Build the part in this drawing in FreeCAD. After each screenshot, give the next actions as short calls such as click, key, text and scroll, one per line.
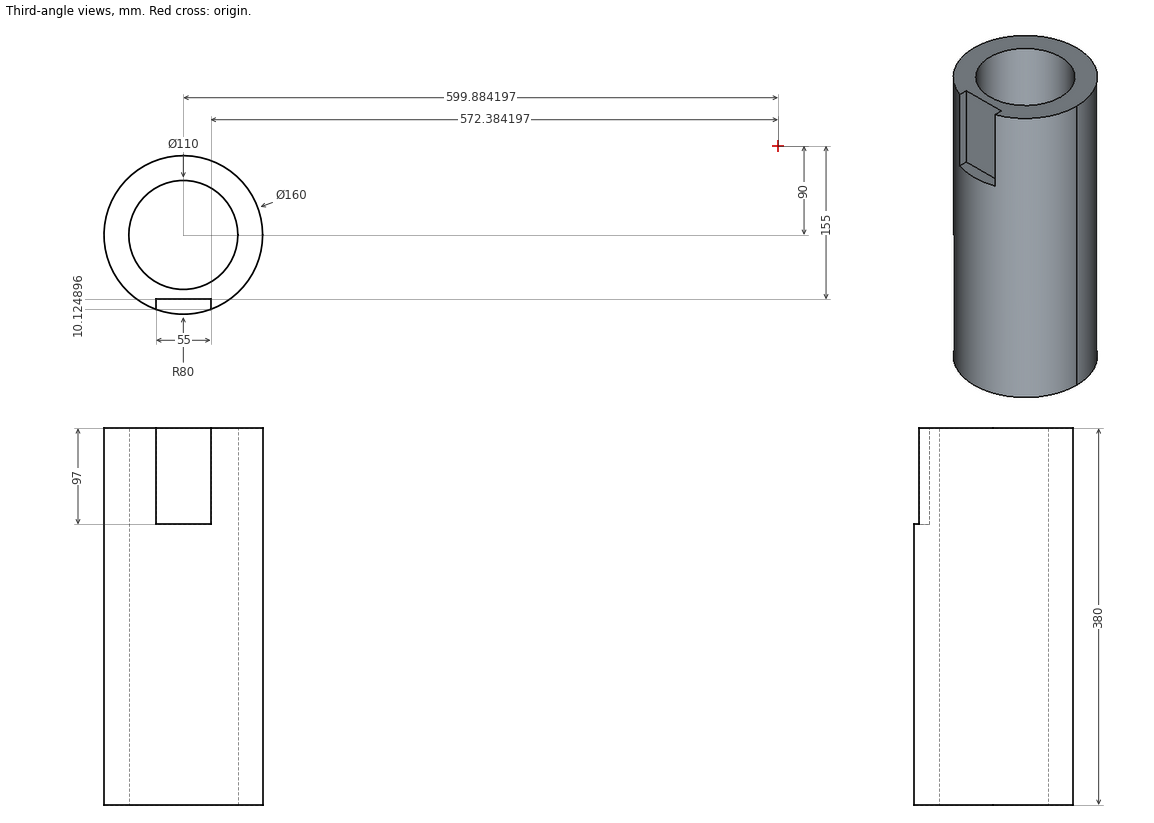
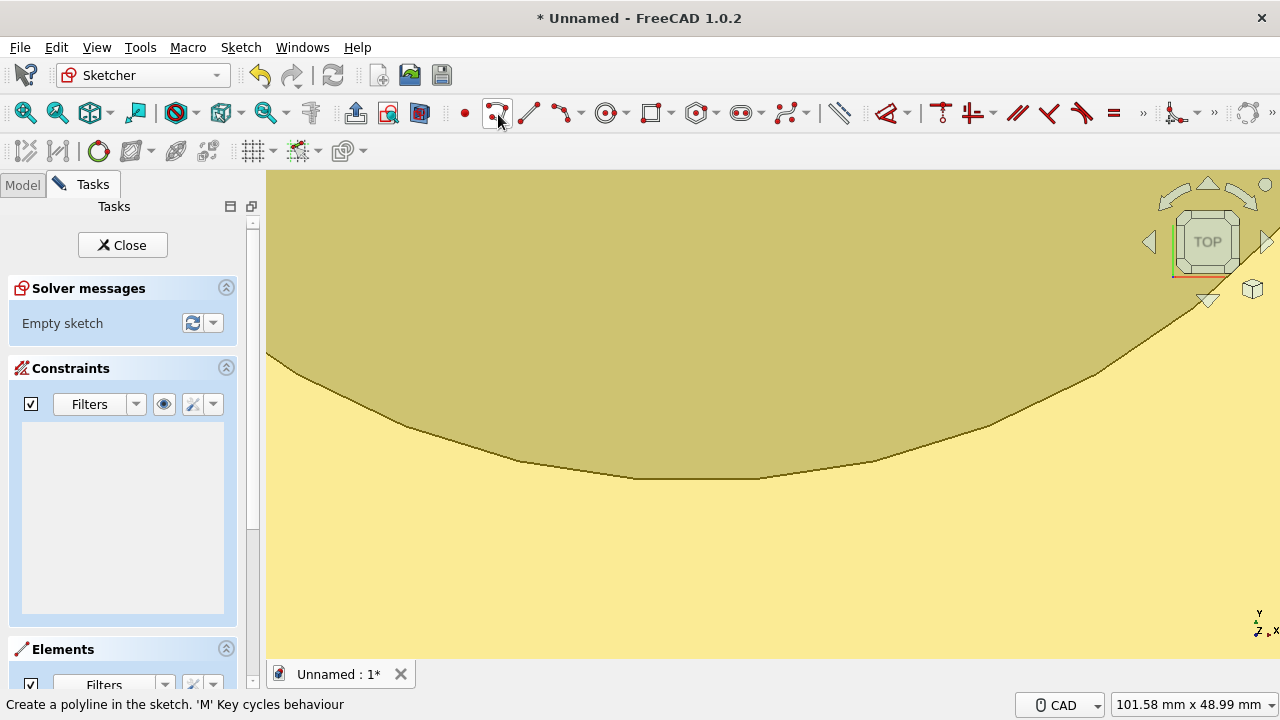
click(971, 433)
click(971, 332)
click(422, 332)
click(422, 433)
right_click(422, 433)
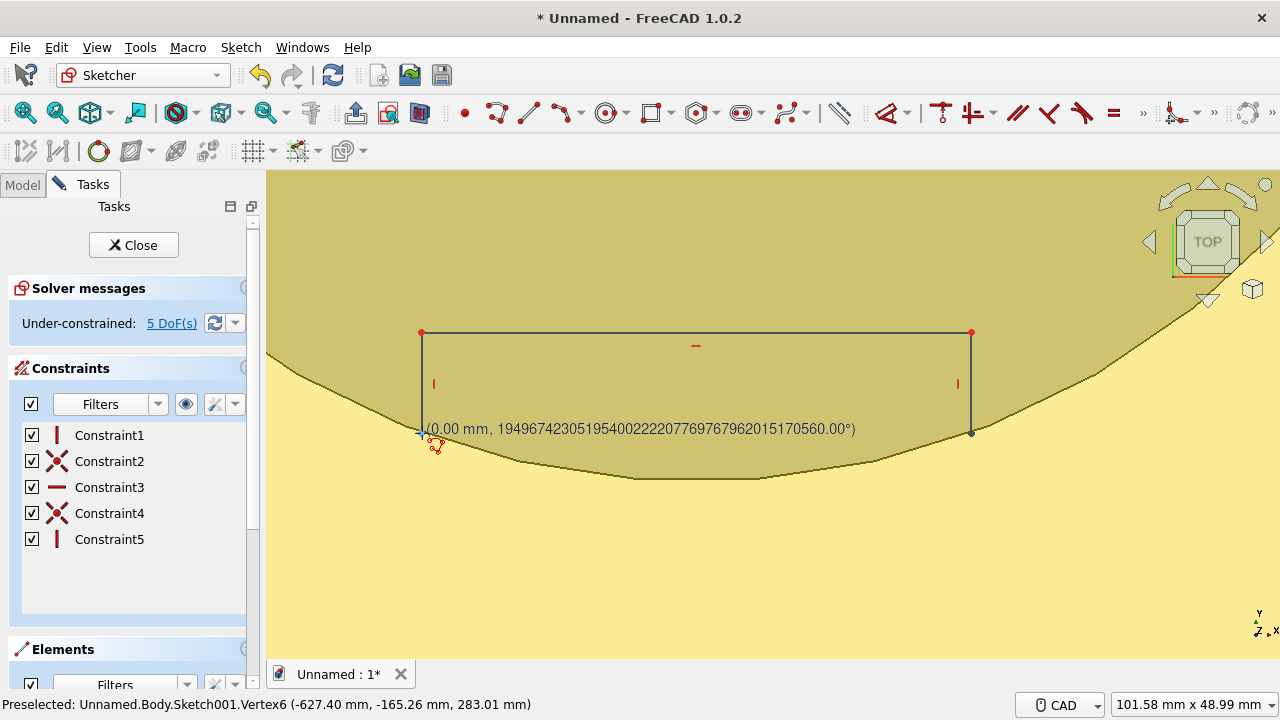
click(562, 114)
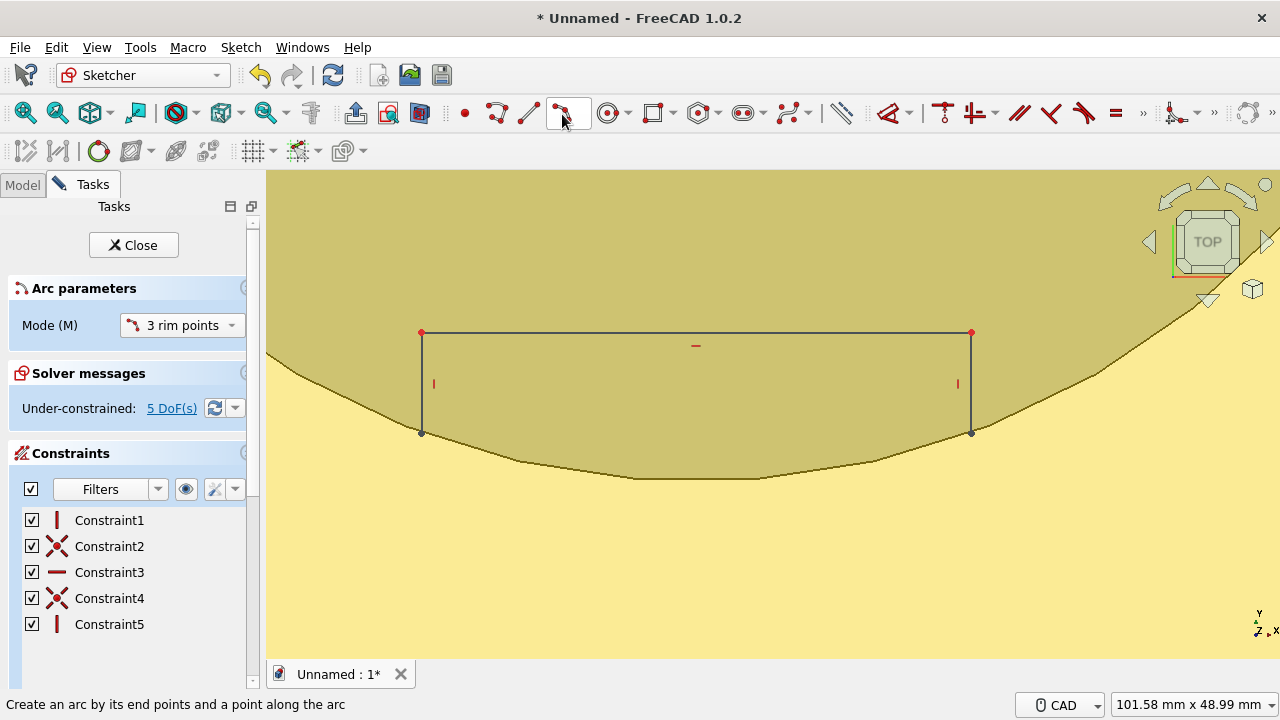
click(422, 434)
click(971, 434)
click(697, 481)
key(Escape)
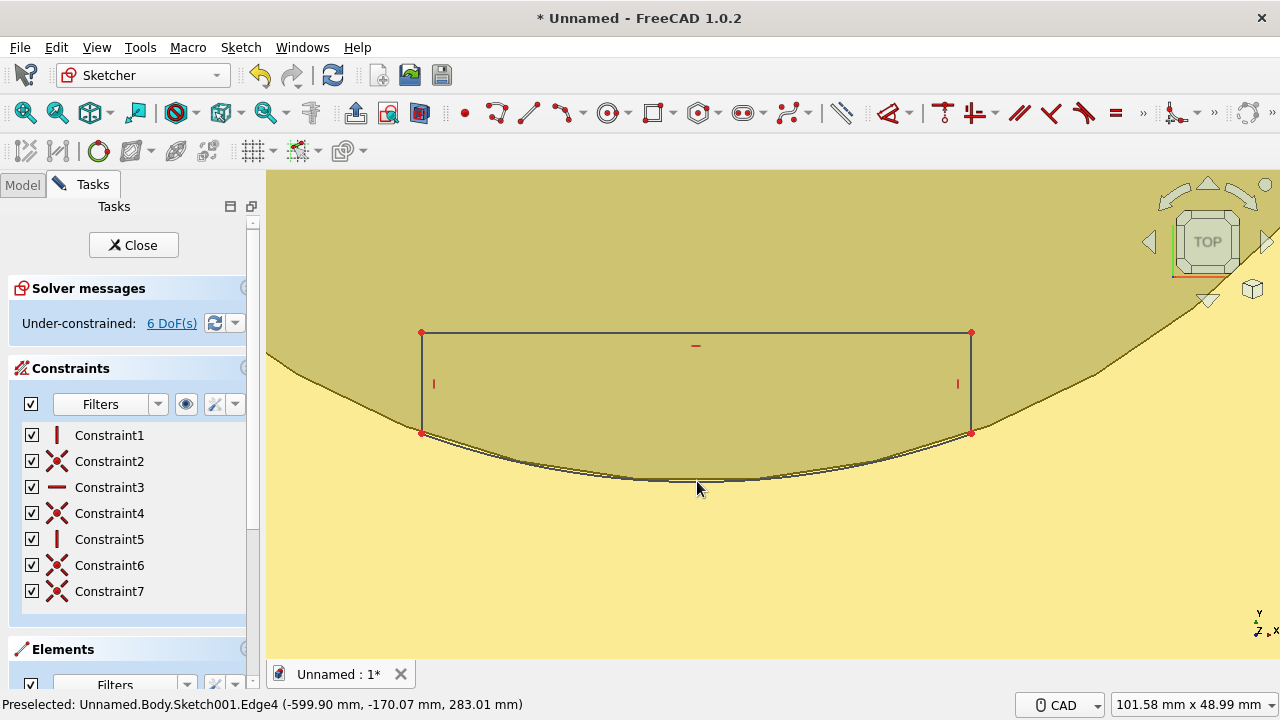
click(888, 114)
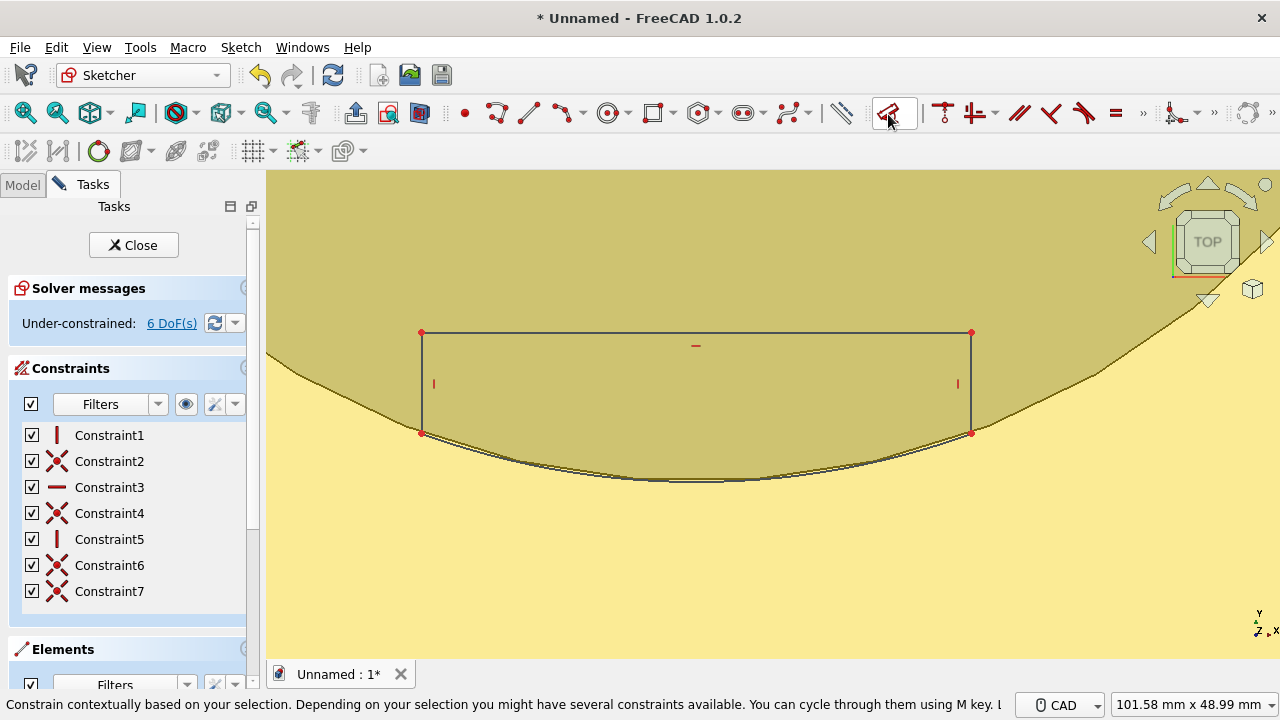
click(585, 474)
click(581, 506)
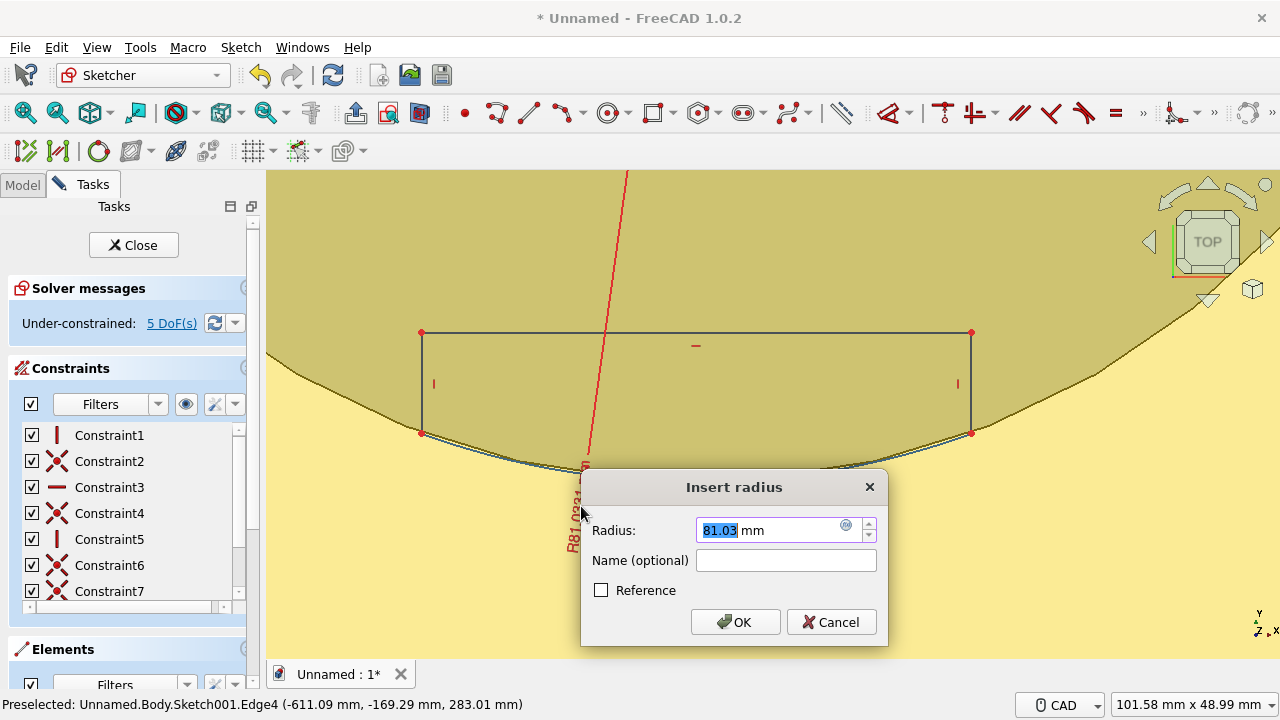
text(80)
key(Return)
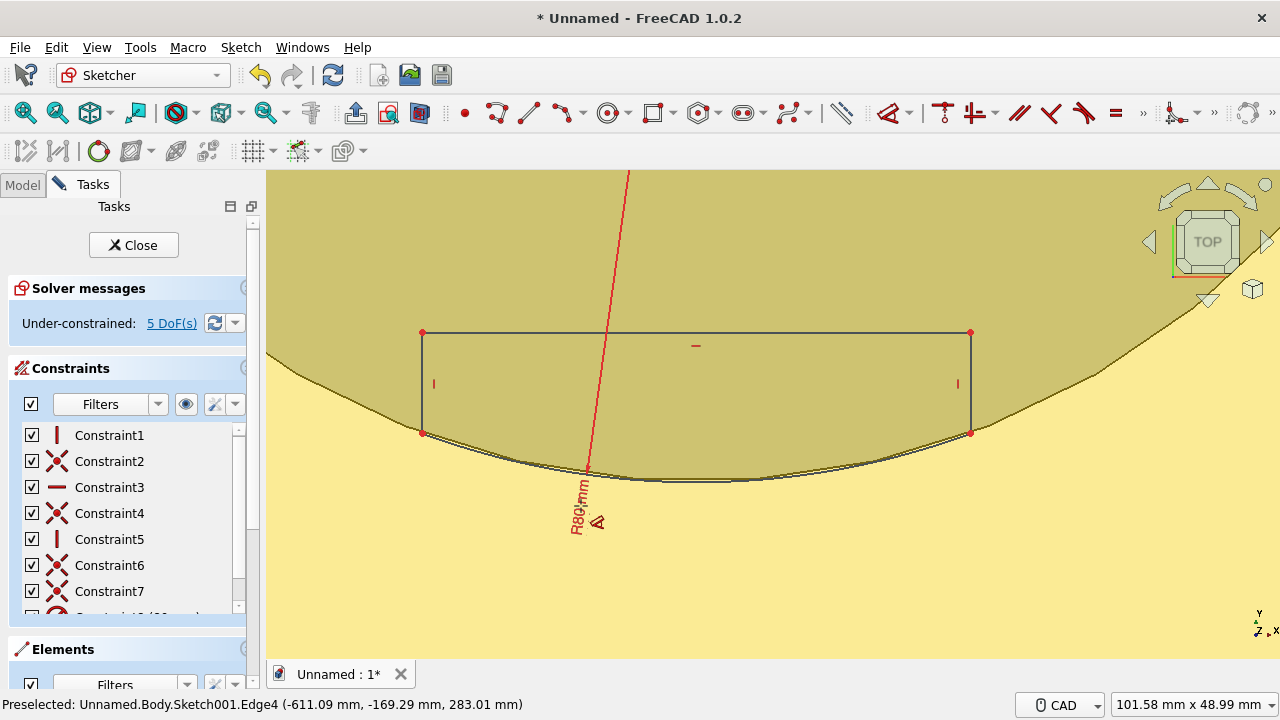
click(806, 333)
click(696, 299)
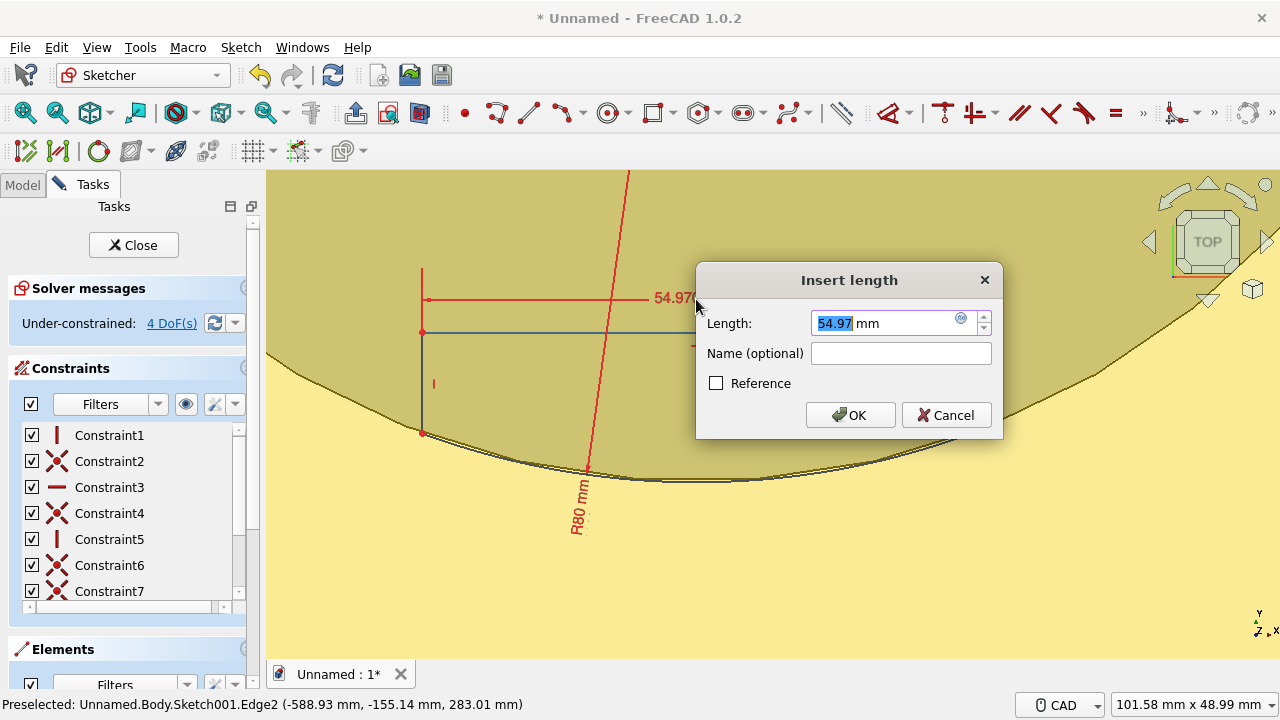
text(55)
key(Return)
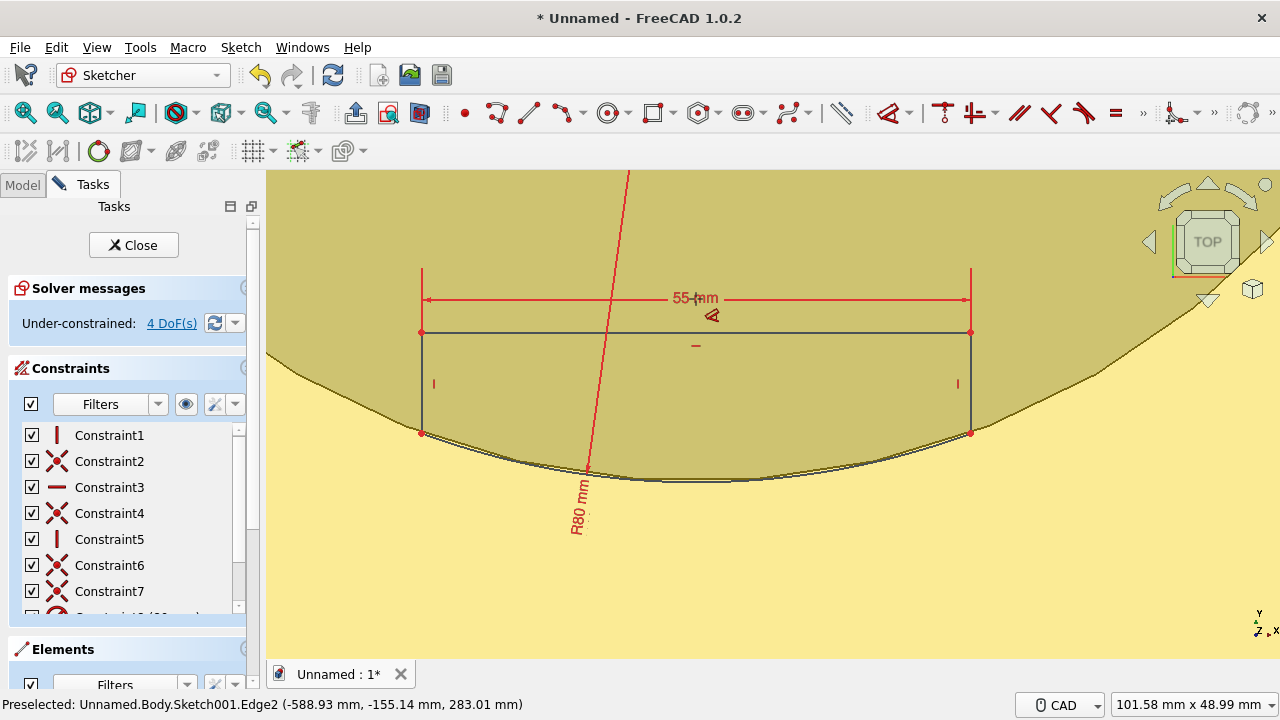
scroll(709, 608, down, 5)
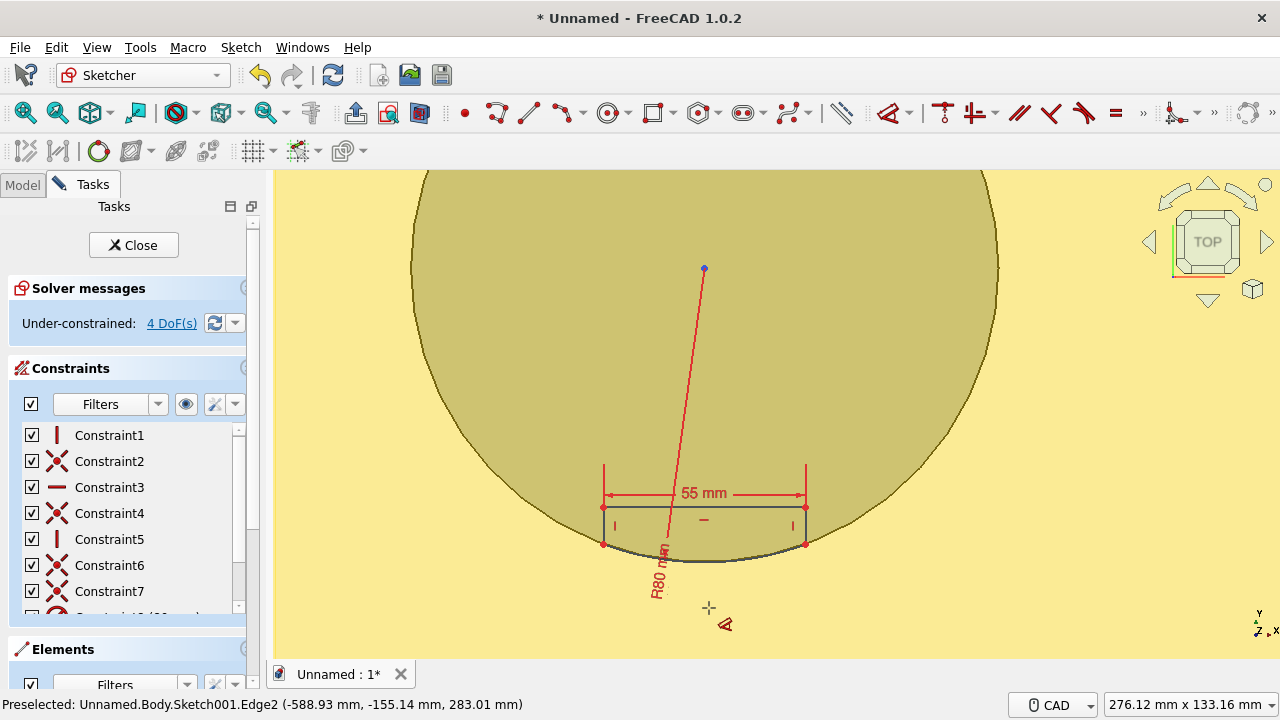
click(705, 269)
click(671, 233)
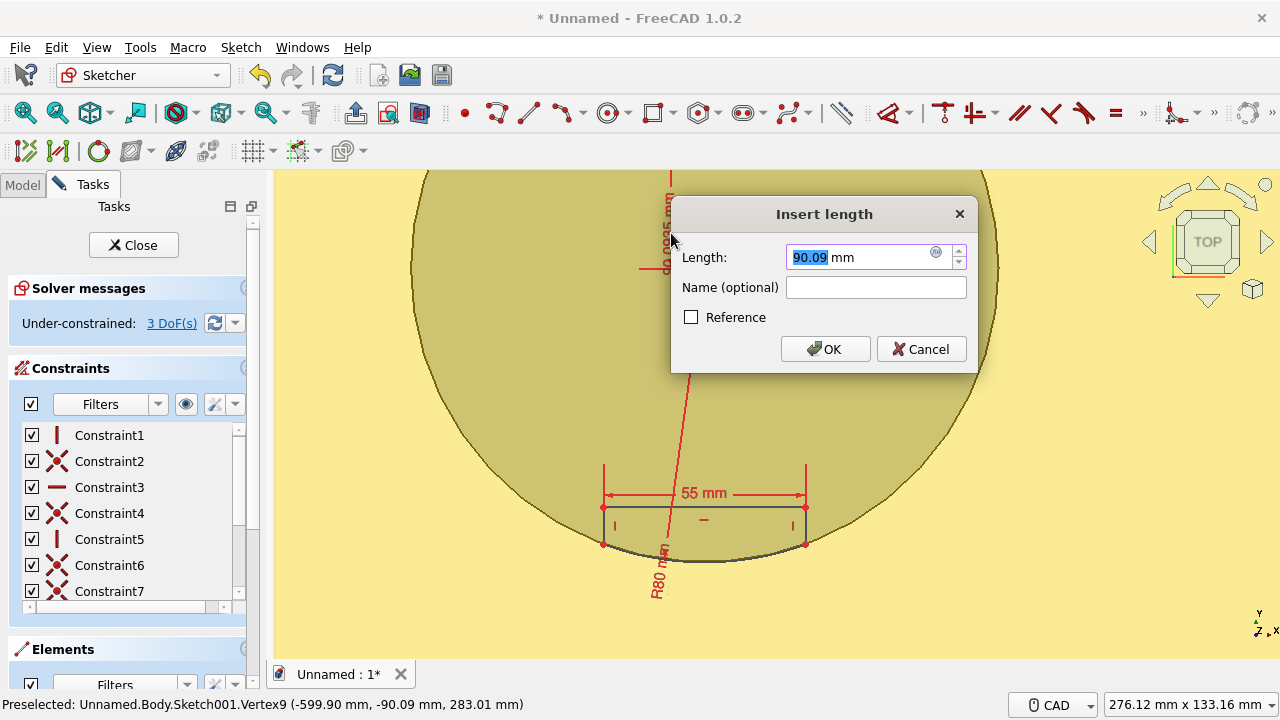
text(90)
key(Return)